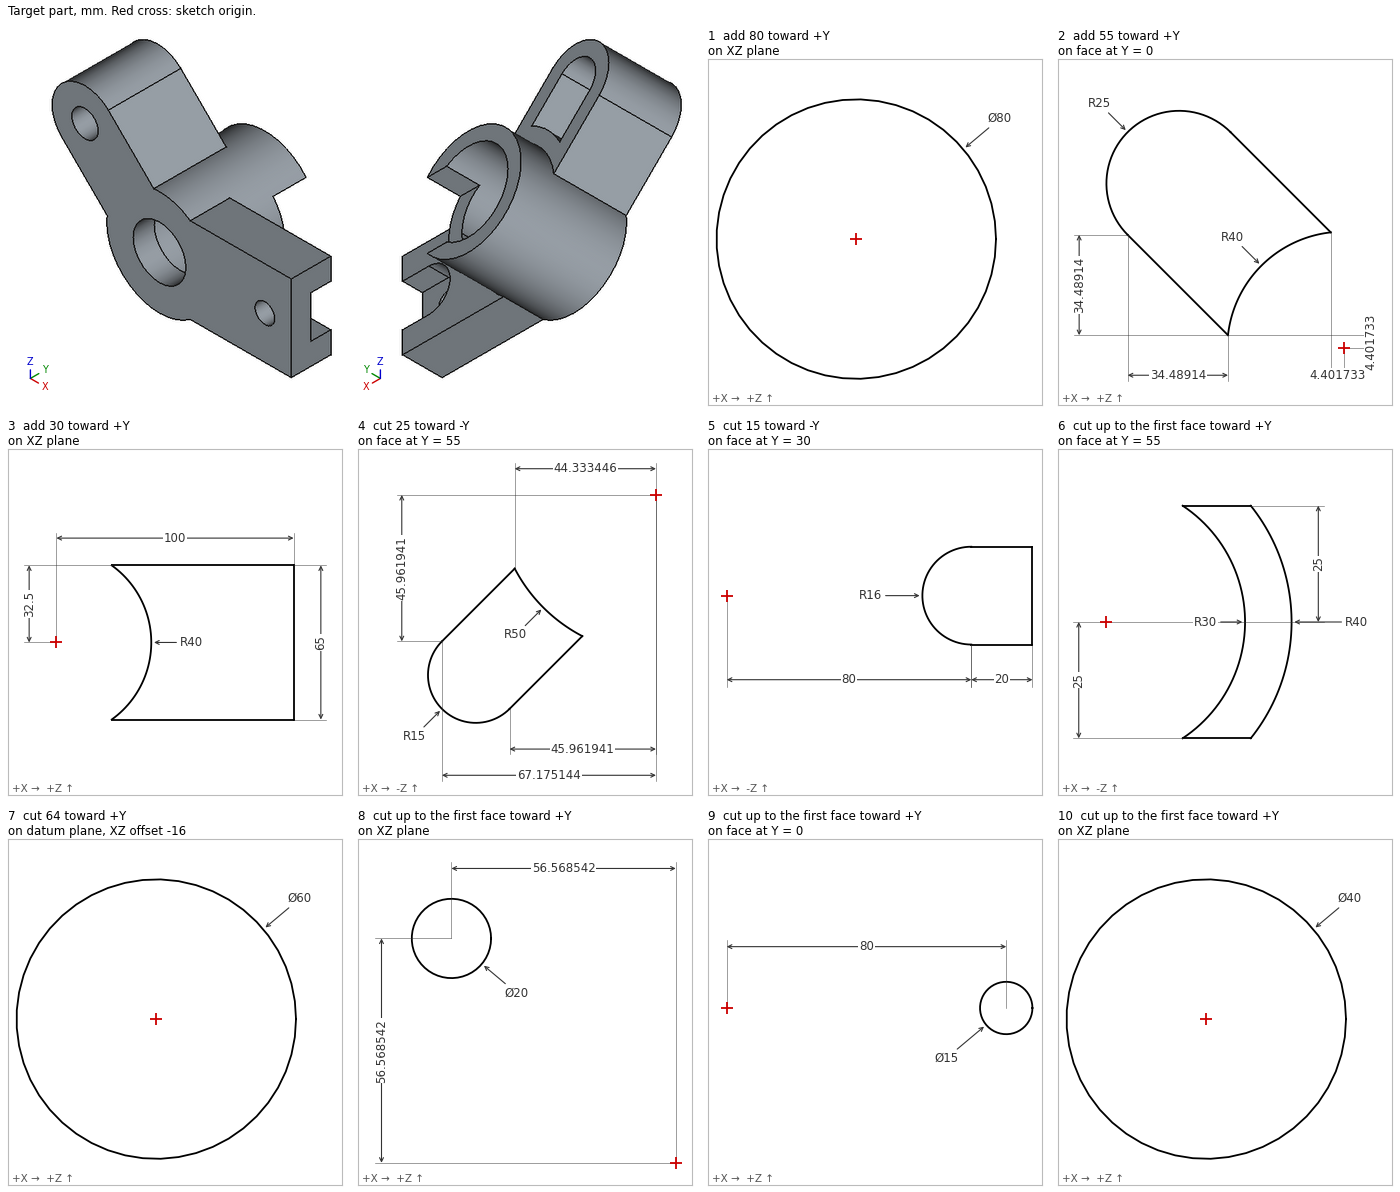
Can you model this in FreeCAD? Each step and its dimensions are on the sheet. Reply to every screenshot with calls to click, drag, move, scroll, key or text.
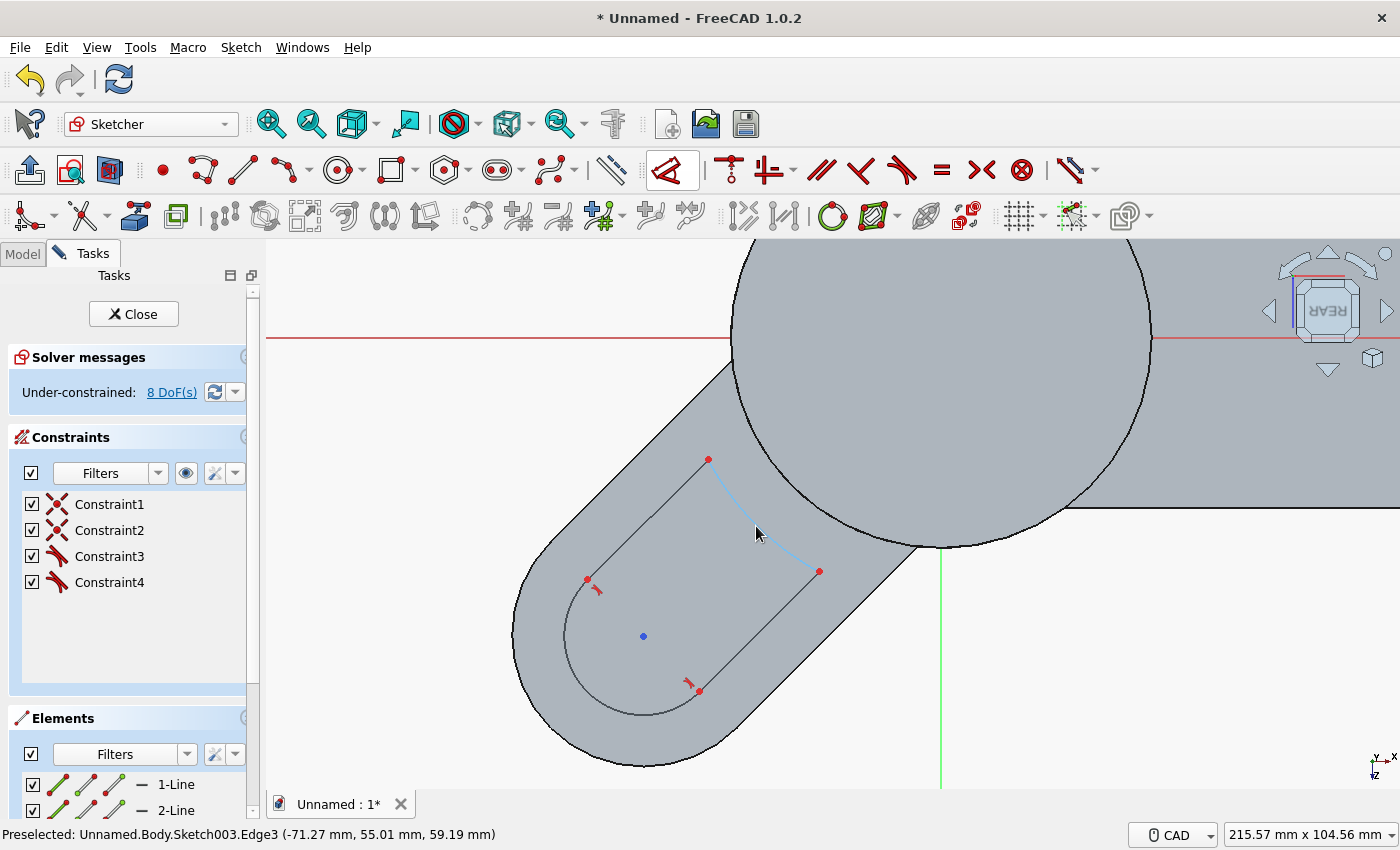
drag(931, 323, 959, 348)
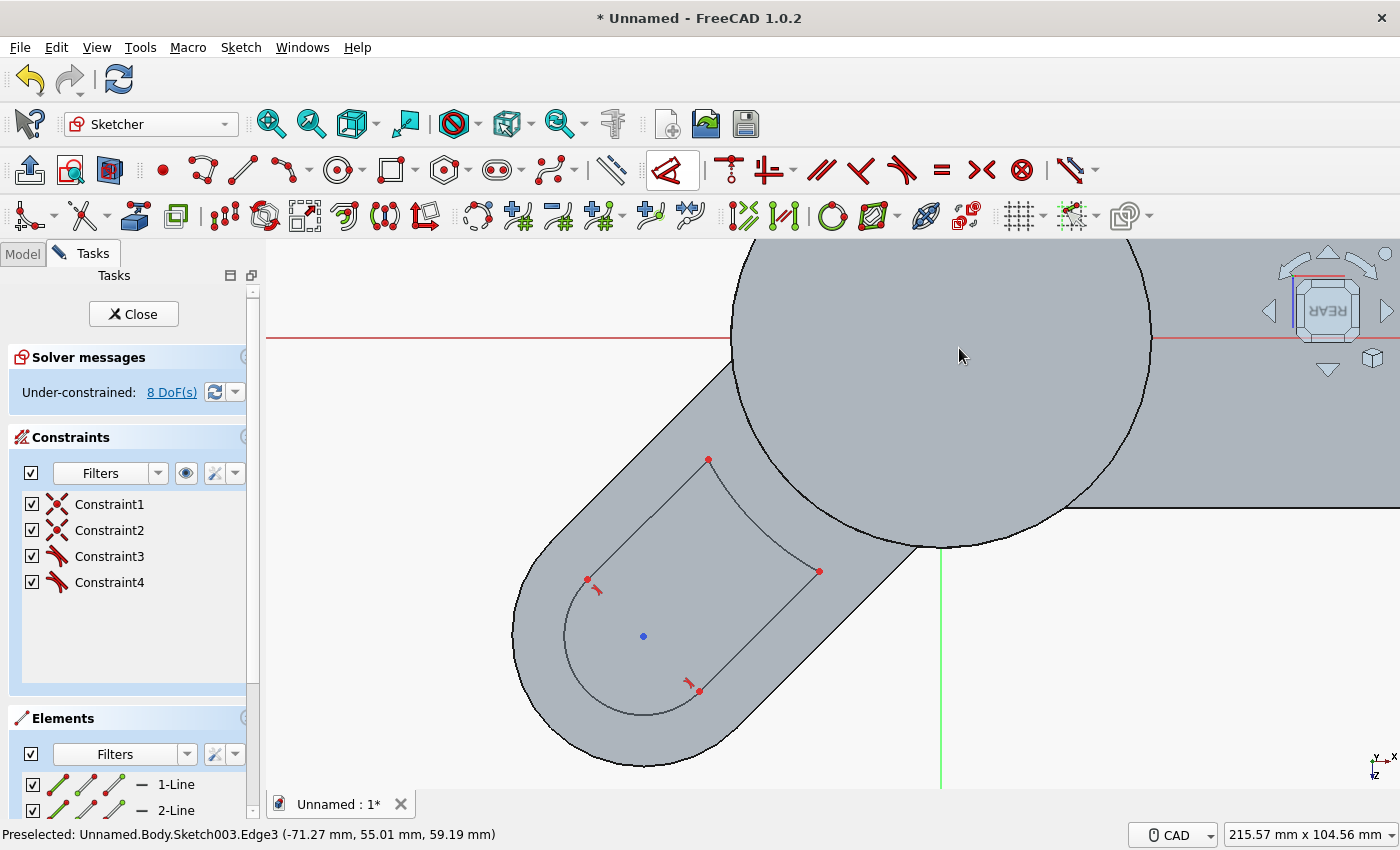
click(730, 170)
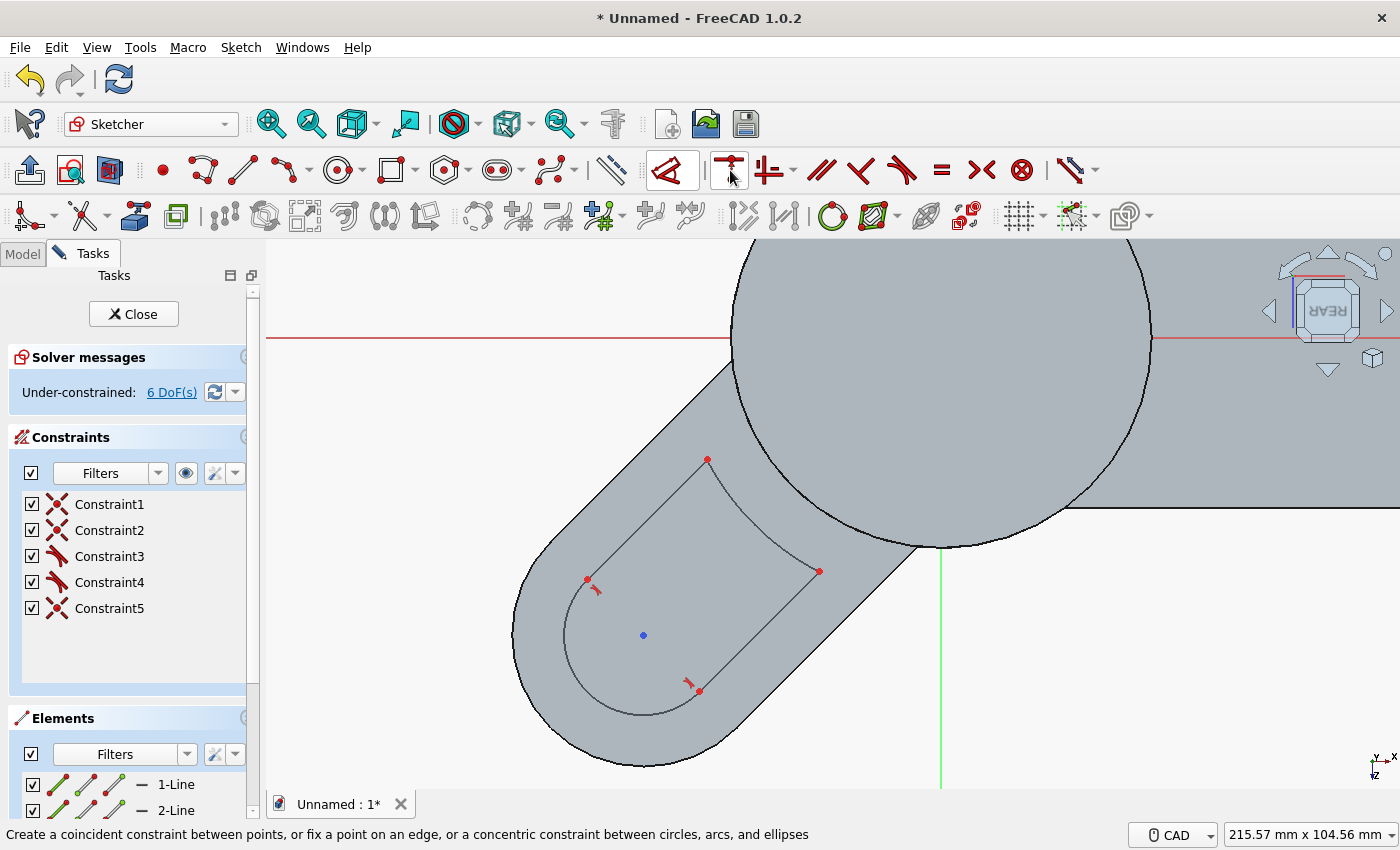
click(565, 648)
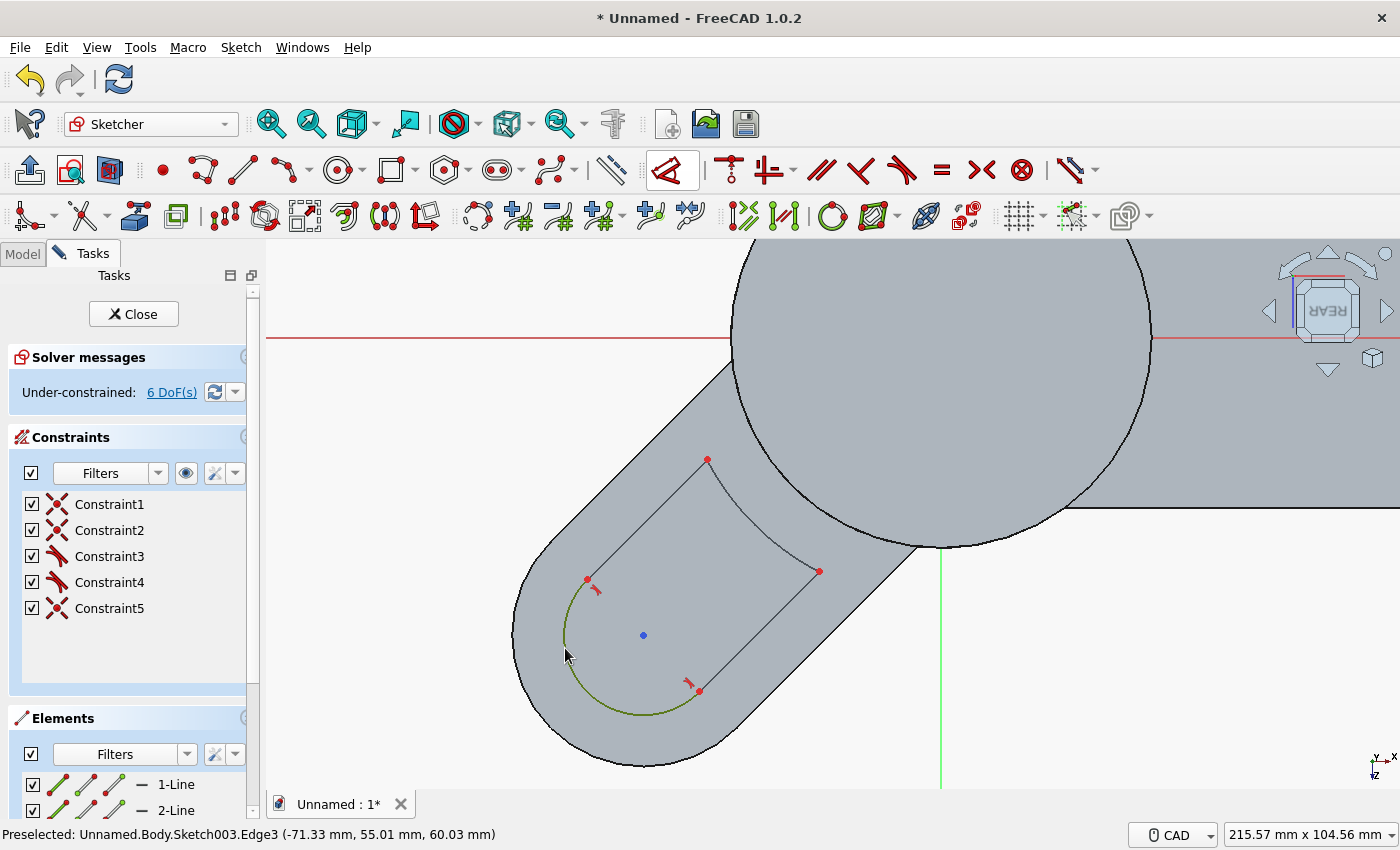
click(694, 170)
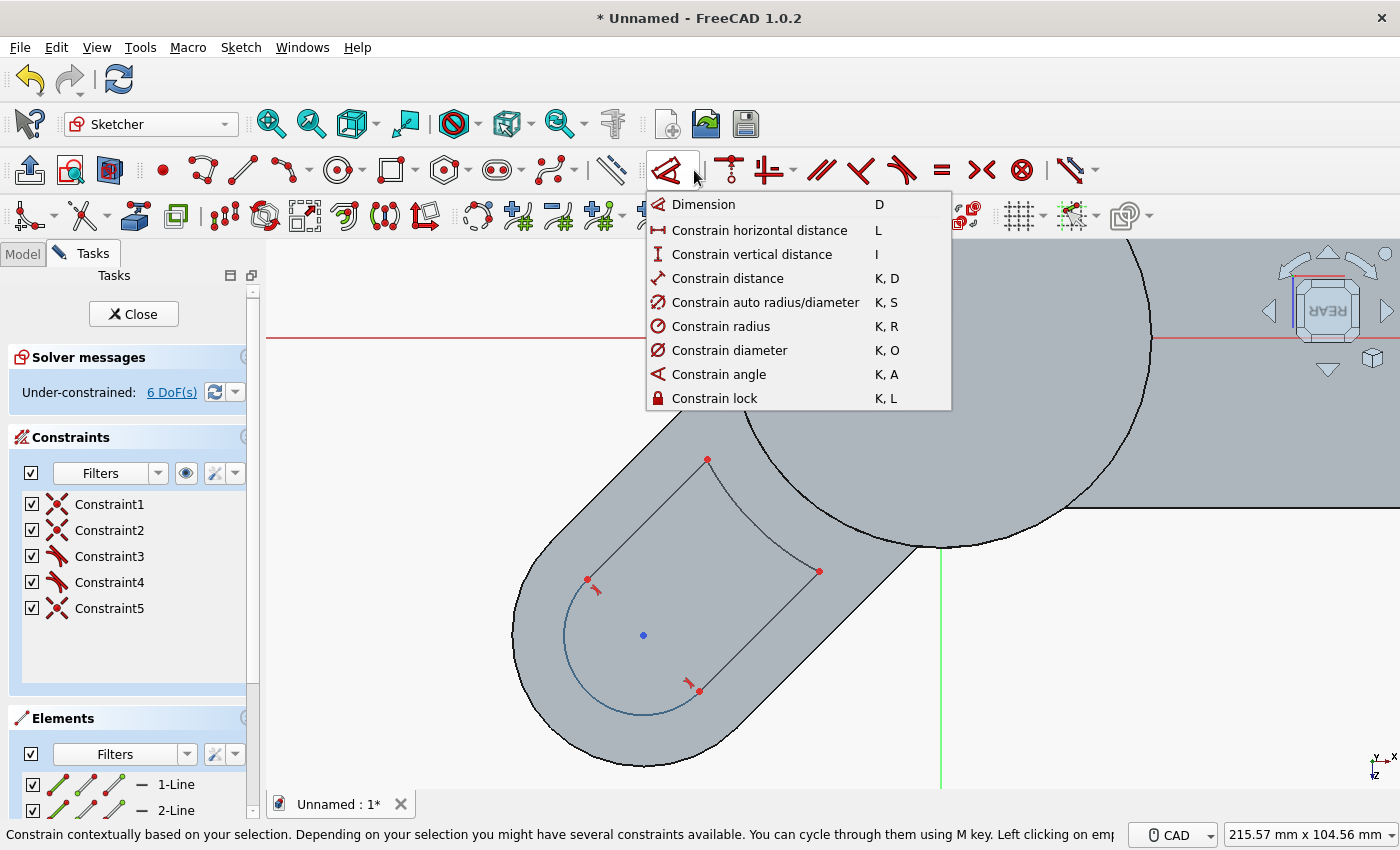
click(799, 326)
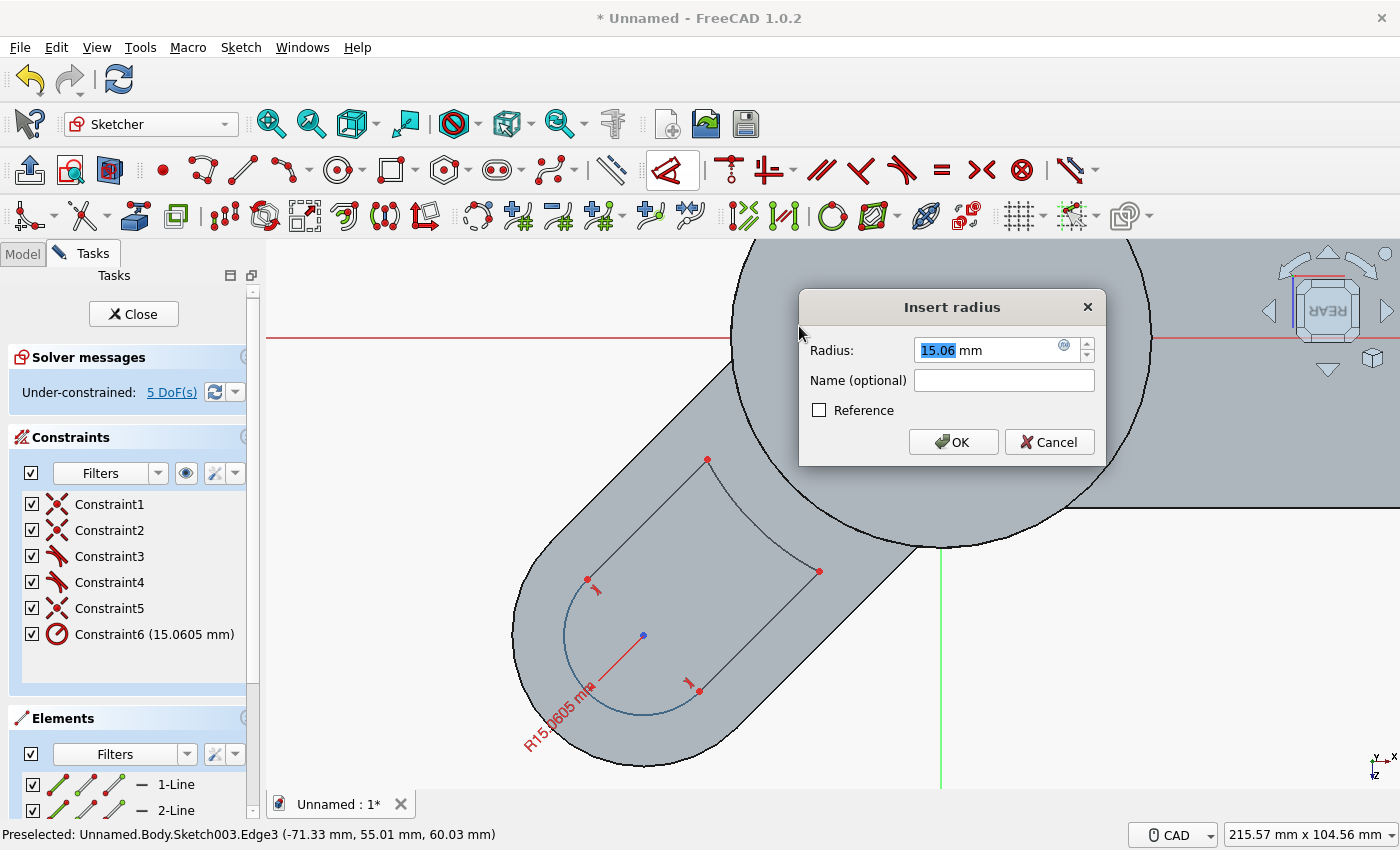
text(15)
key(Return)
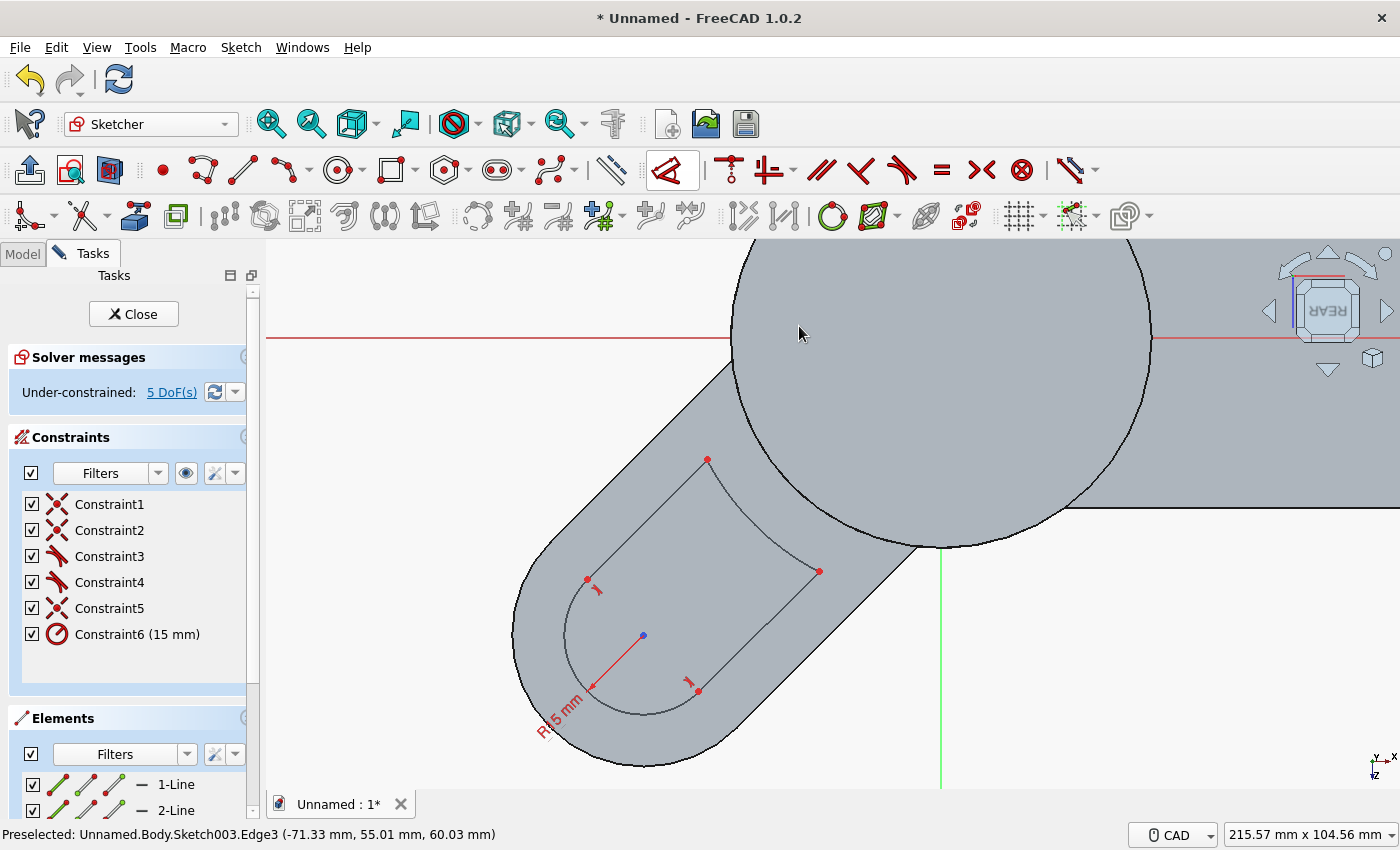
click(733, 501)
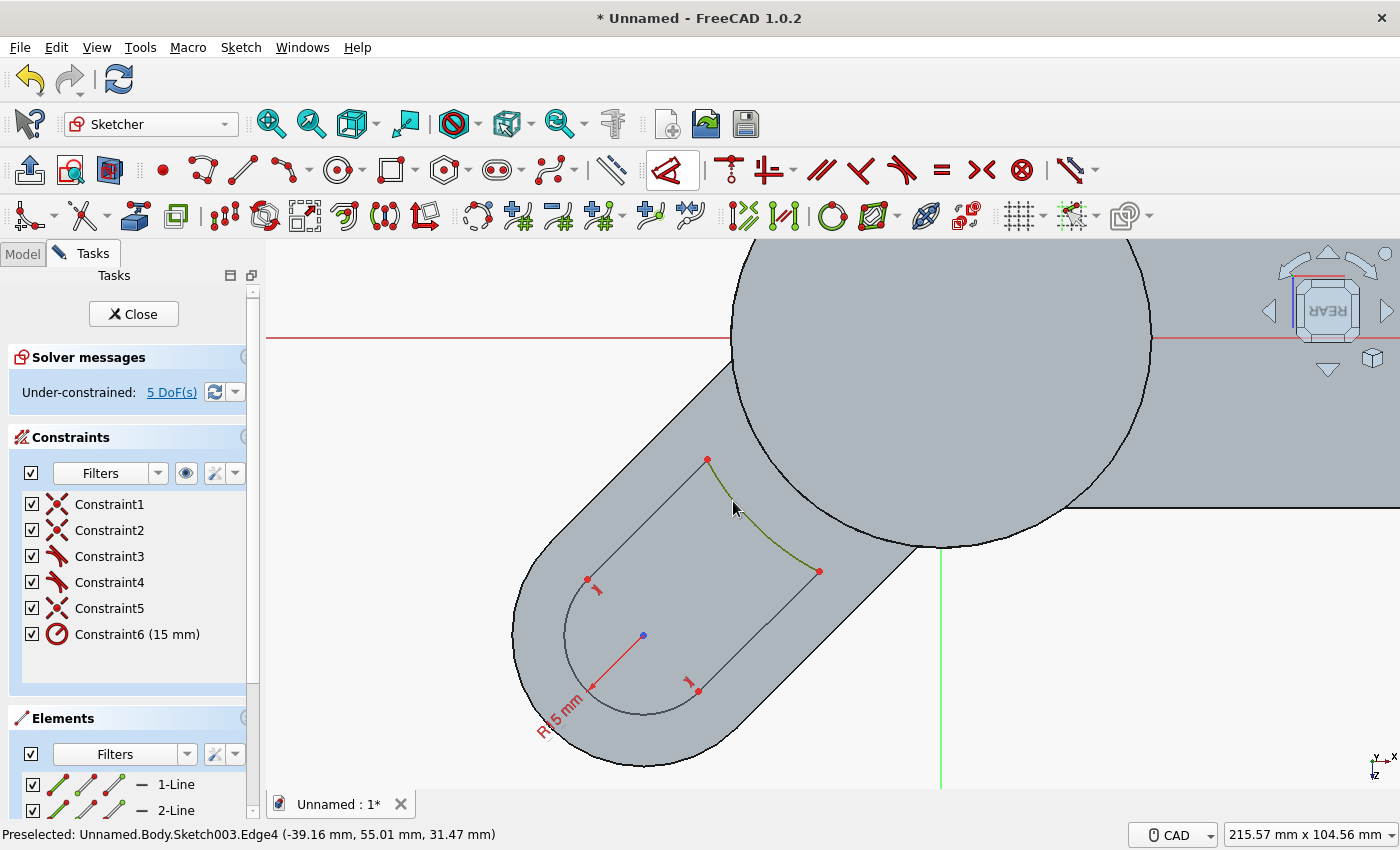
key(k)
key(r)